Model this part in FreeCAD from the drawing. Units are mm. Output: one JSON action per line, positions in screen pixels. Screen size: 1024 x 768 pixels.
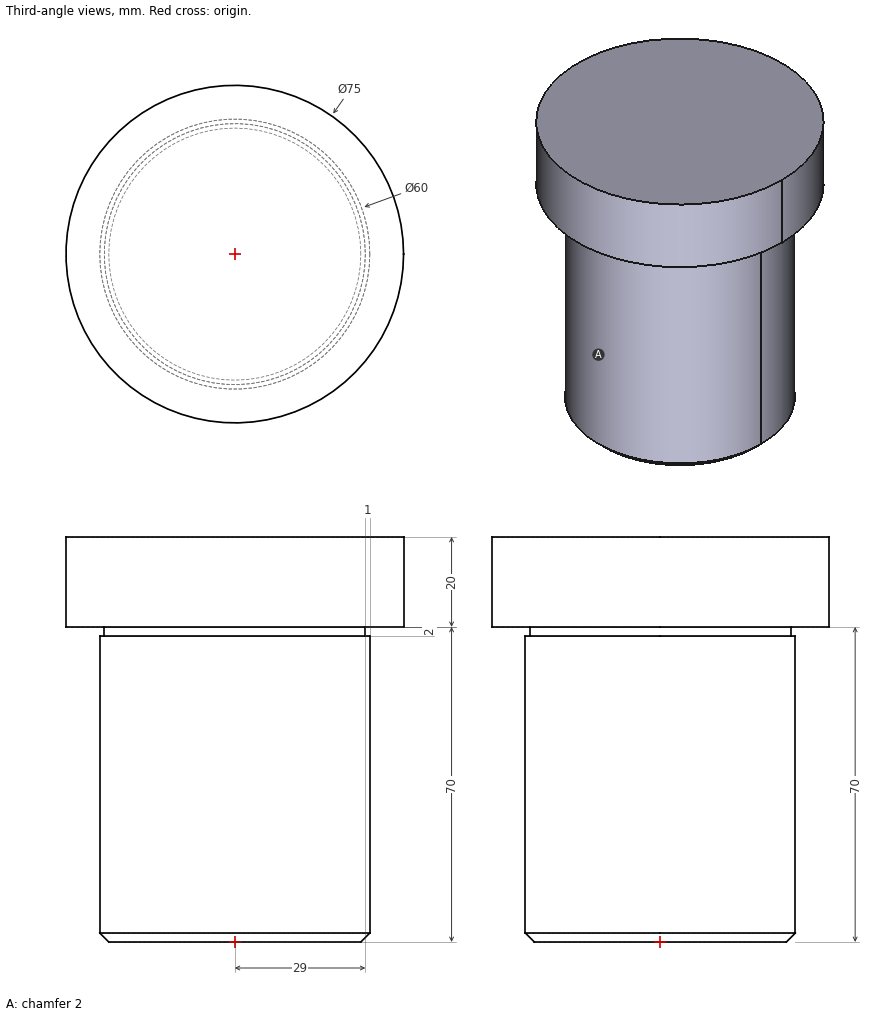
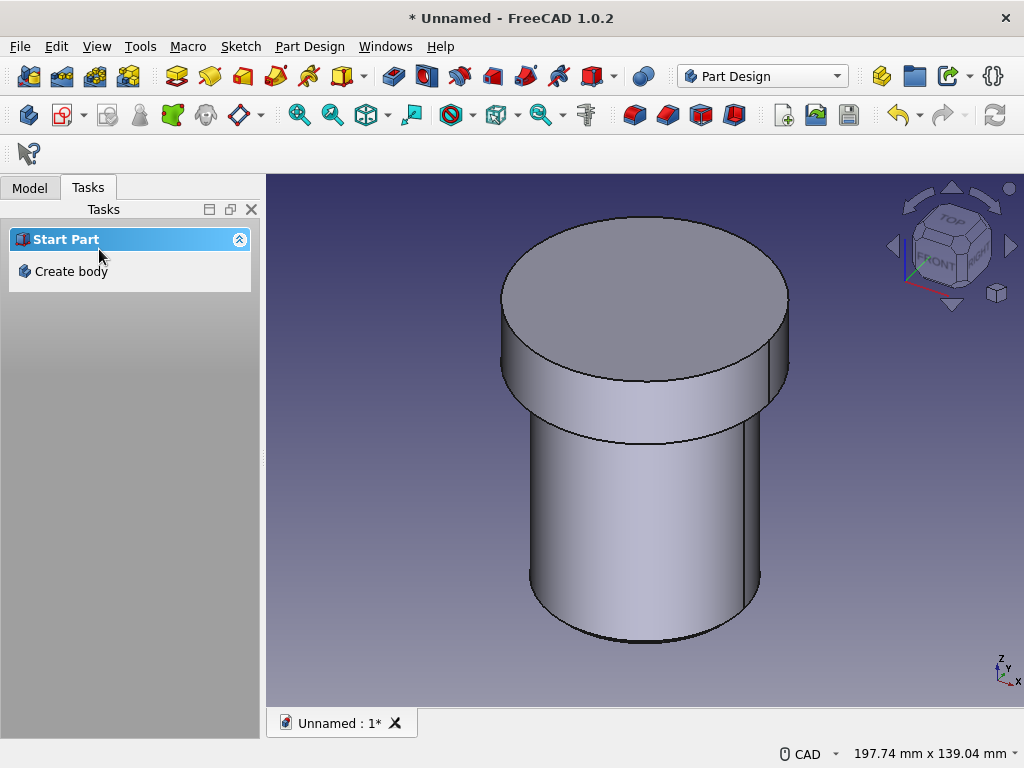
{"action": "left_click", "coordinate": [62, 116]}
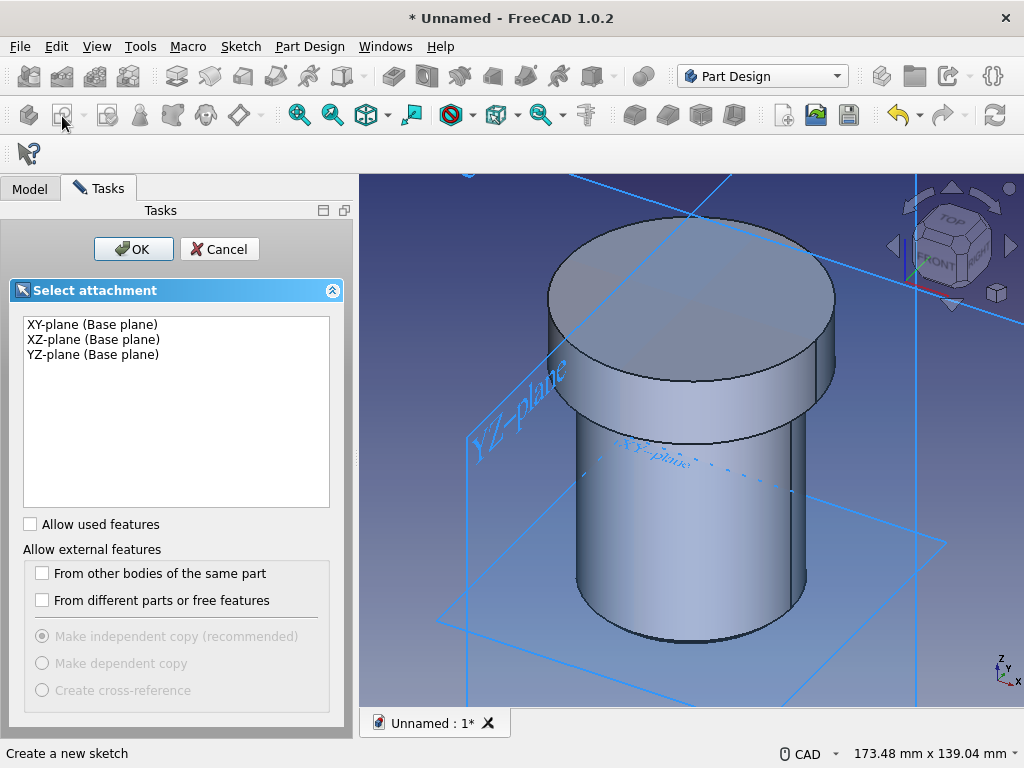
{"action": "left_click", "coordinate": [84, 340]}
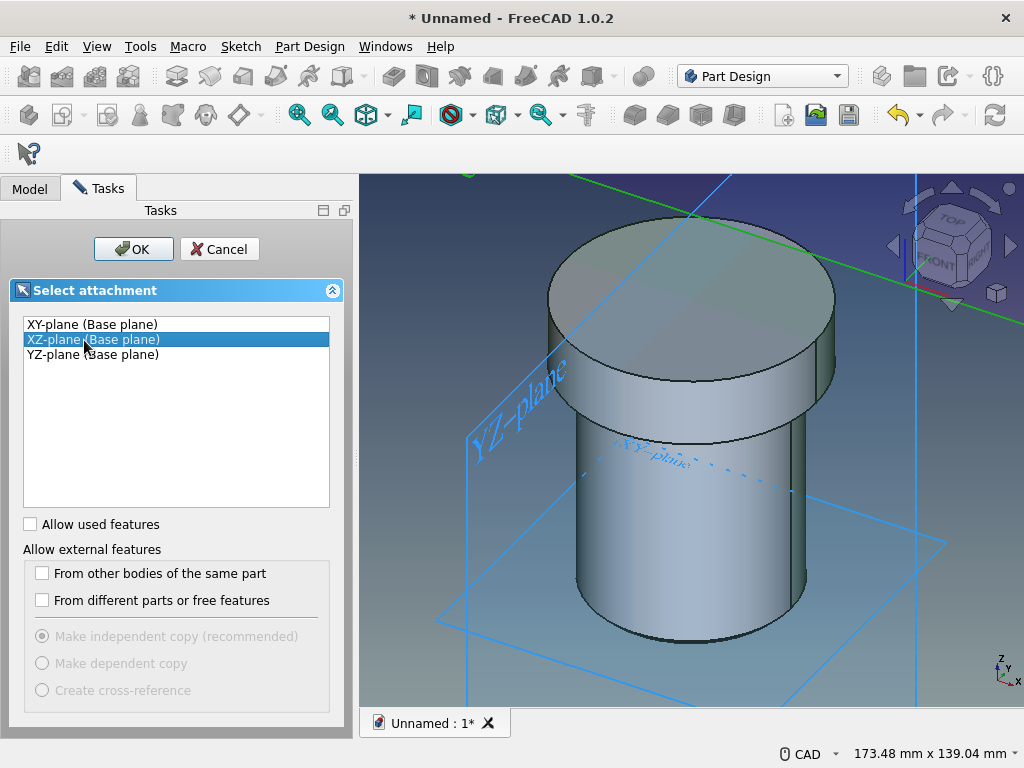
{"action": "left_click", "coordinate": [134, 249]}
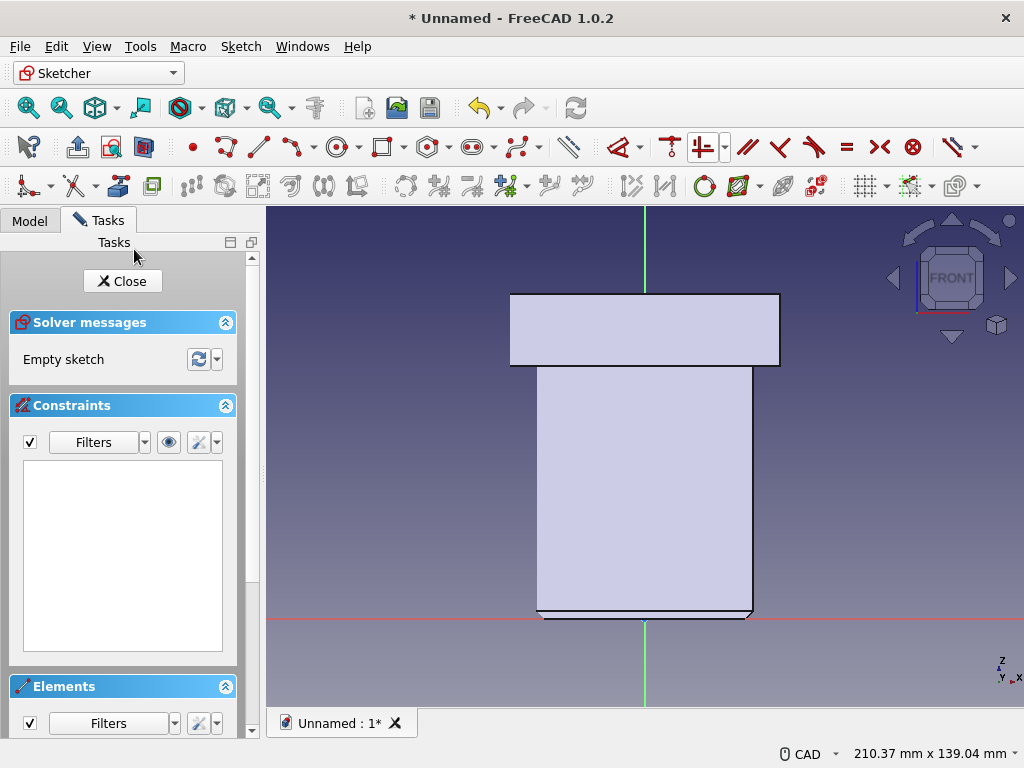
{"action": "left_click", "coordinate": [144, 148]}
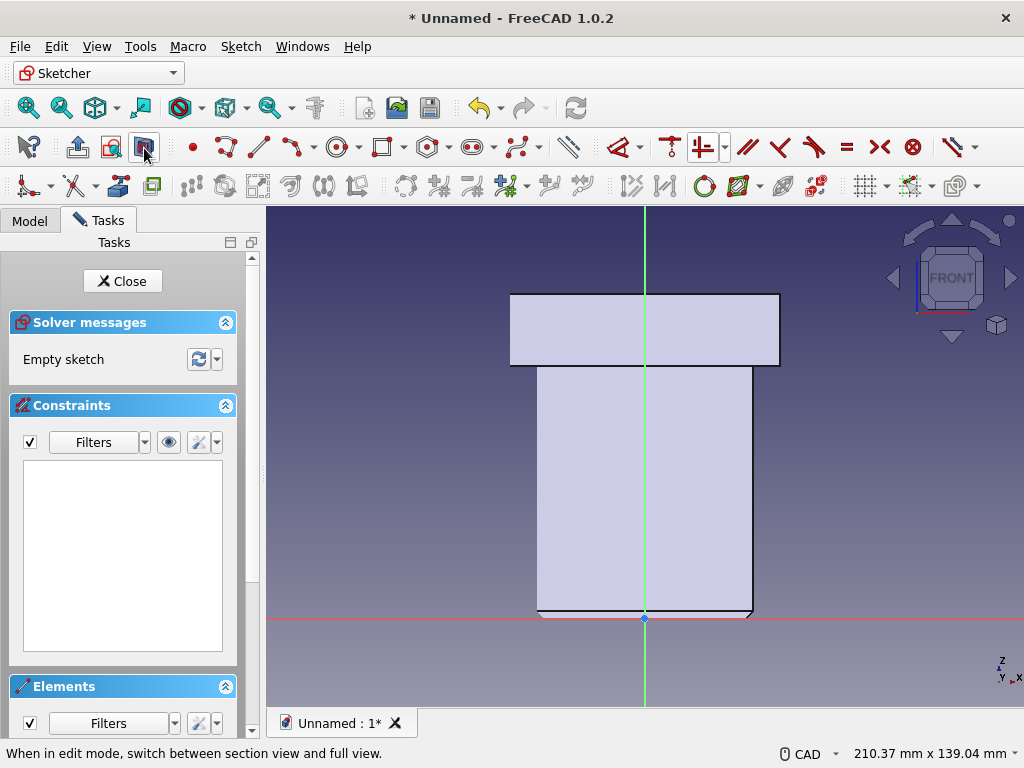
{"action": "scroll", "coordinate": [760, 365], "scroll_direction": "up", "scroll_amount": 15}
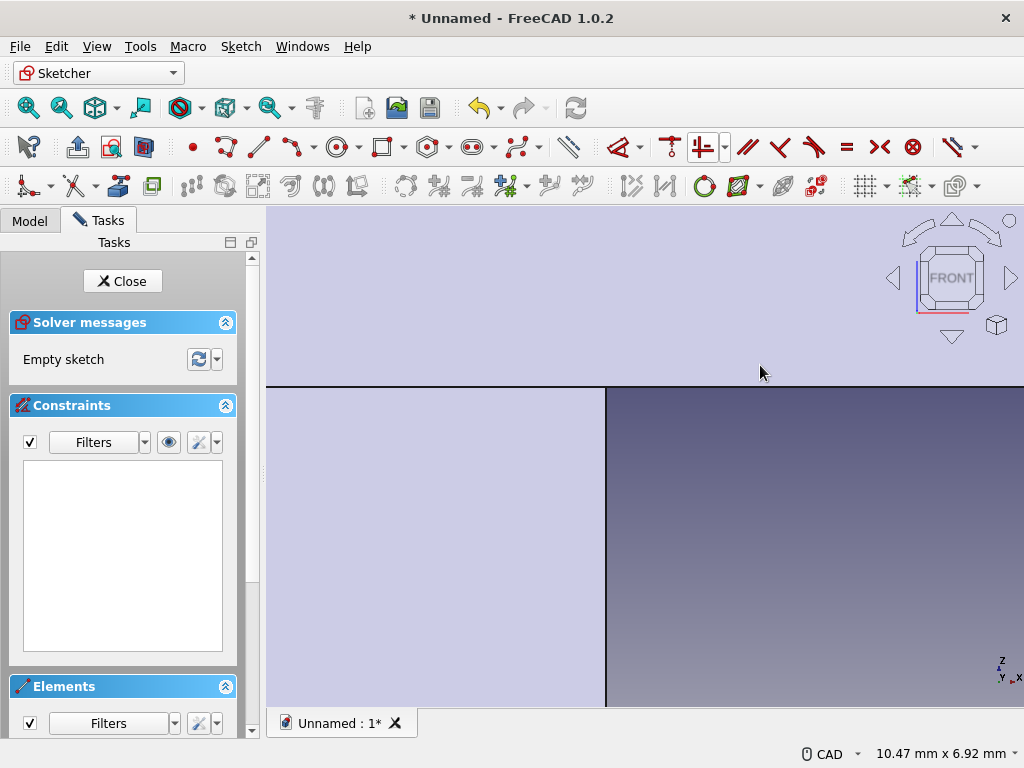
{"action": "scroll", "coordinate": [565, 463], "scroll_direction": "up", "scroll_amount": 4}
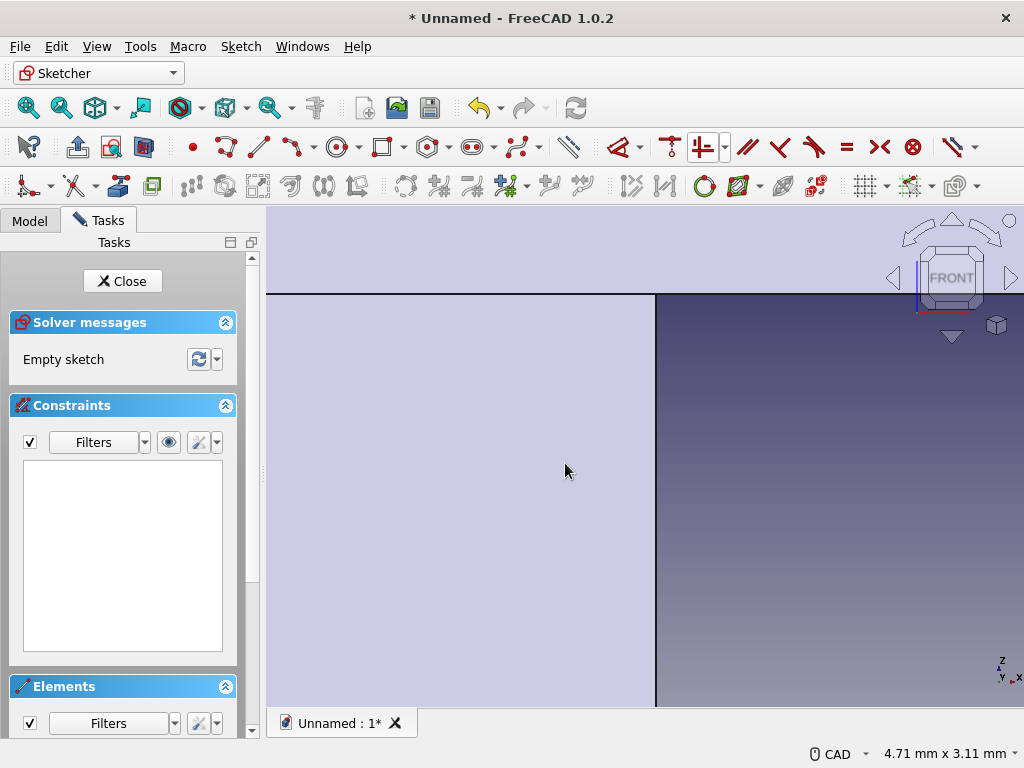
{"action": "key", "text": "g r"}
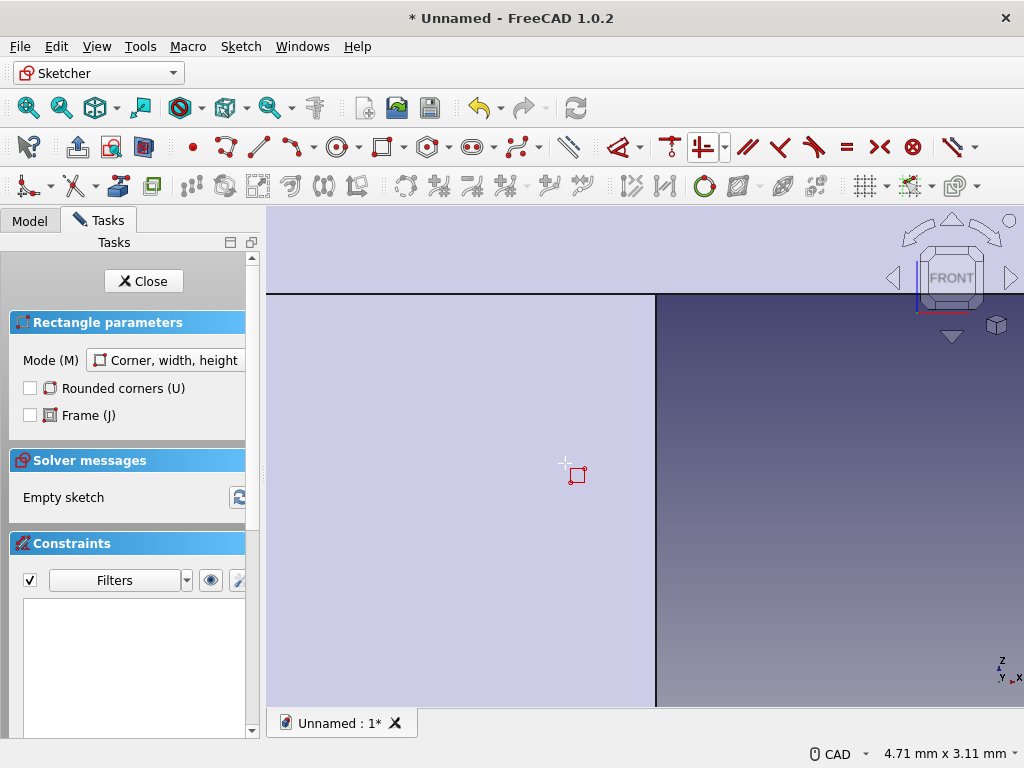
{"action": "left_click", "coordinate": [495, 294]}
{"action": "mouse_move", "coordinate": [656, 616]}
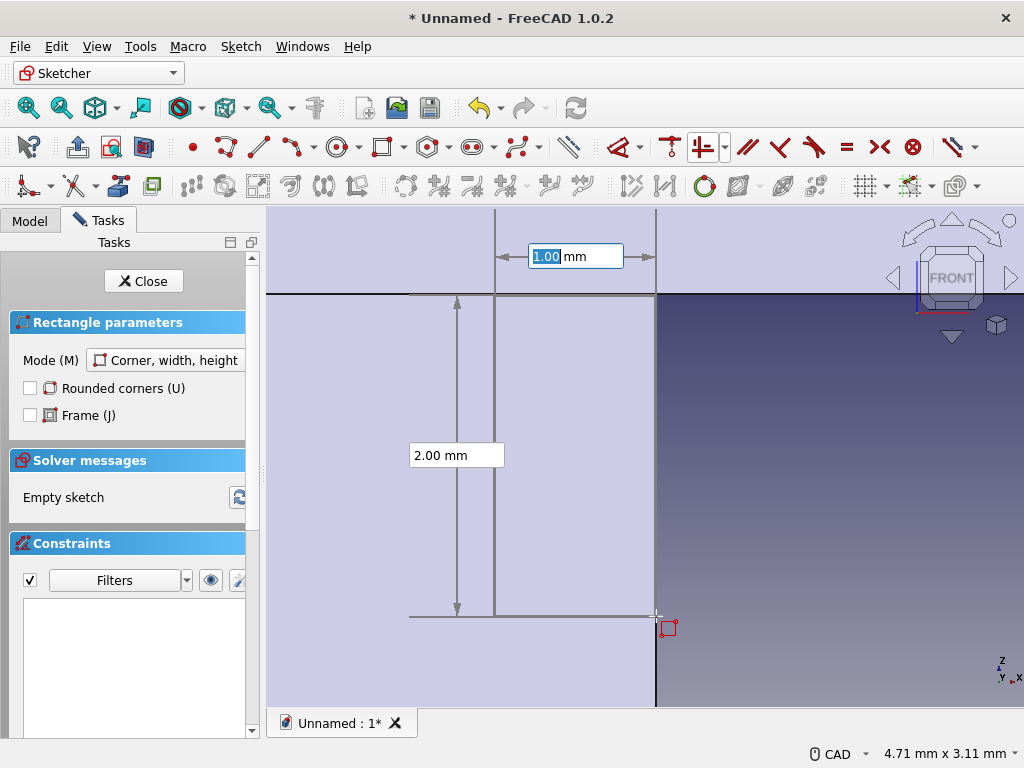
{"action": "type", "text": "1"}
{"action": "key", "text": "Tab"}
{"action": "type", "text": "2"}
{"action": "key", "text": "Return"}
{"action": "key", "text": "Escape"}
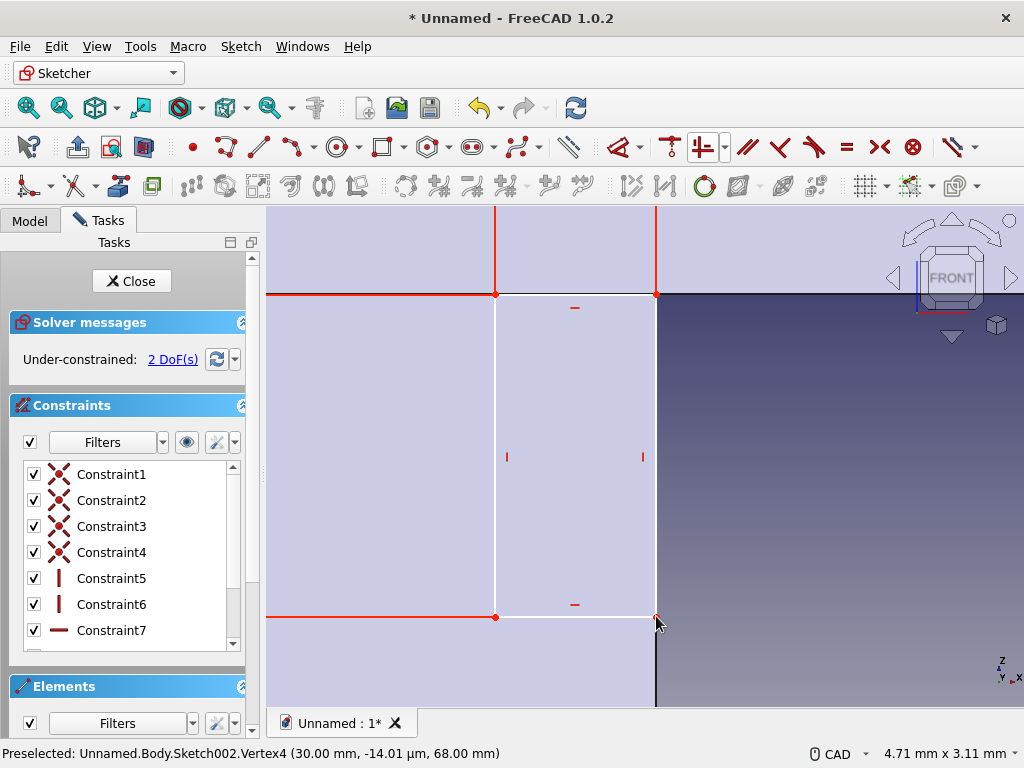
{"action": "left_click", "coordinate": [495, 295]}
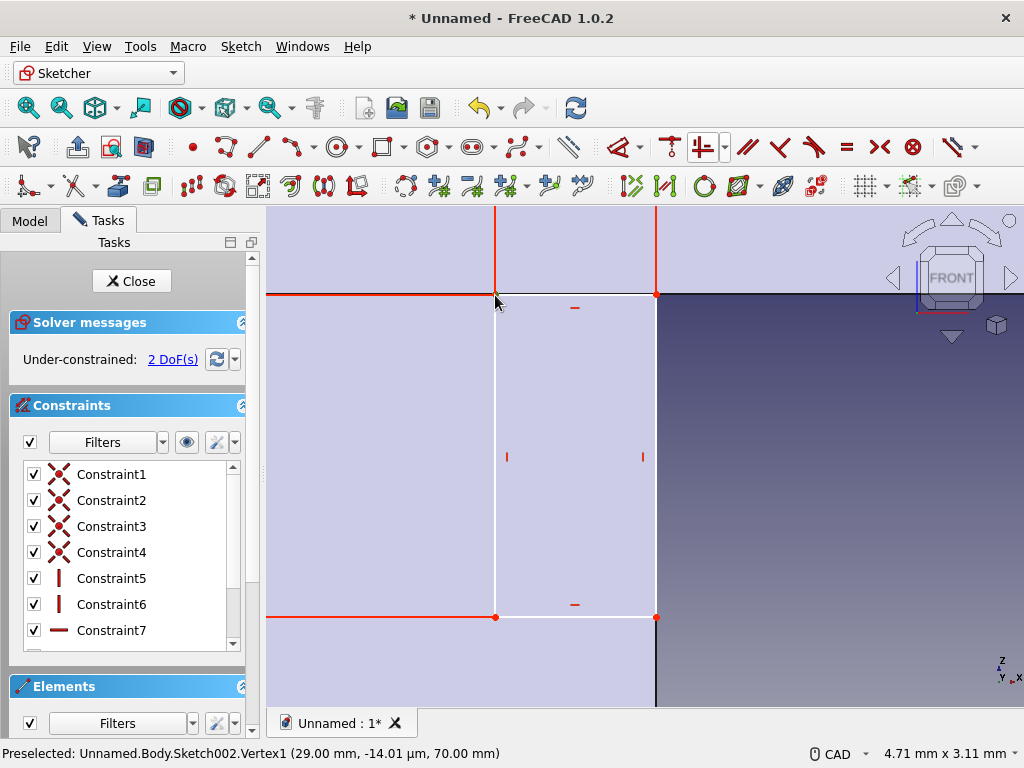
{"action": "key", "text": "l"}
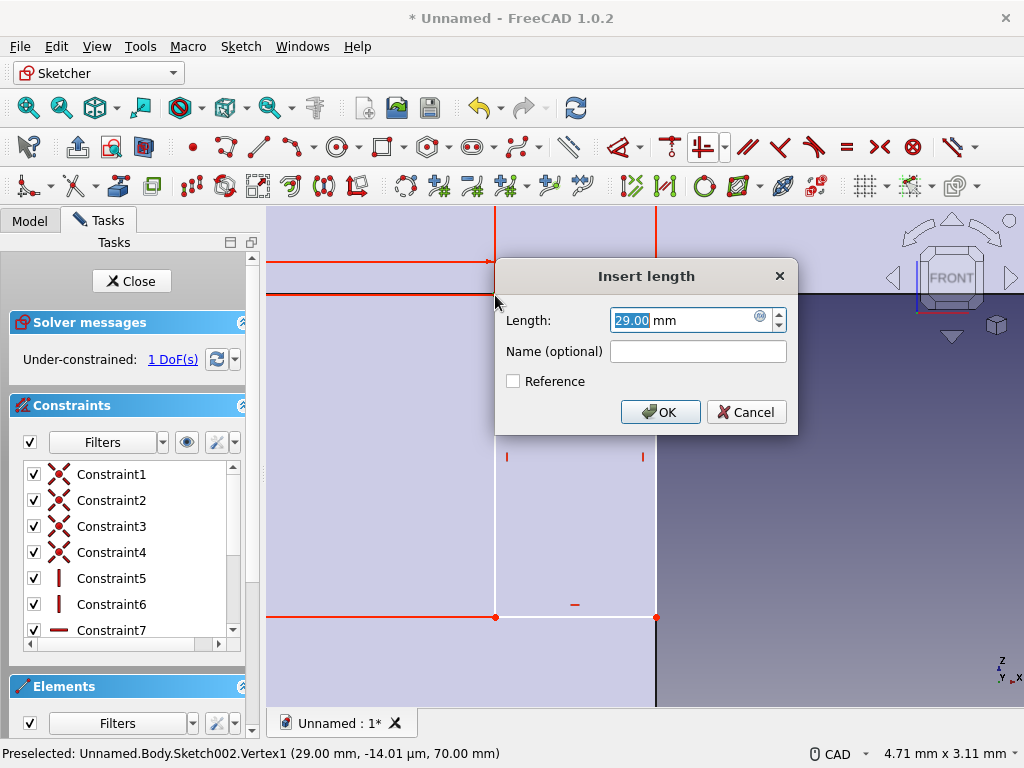
{"action": "type", "text": "29"}
{"action": "key", "text": "Return"}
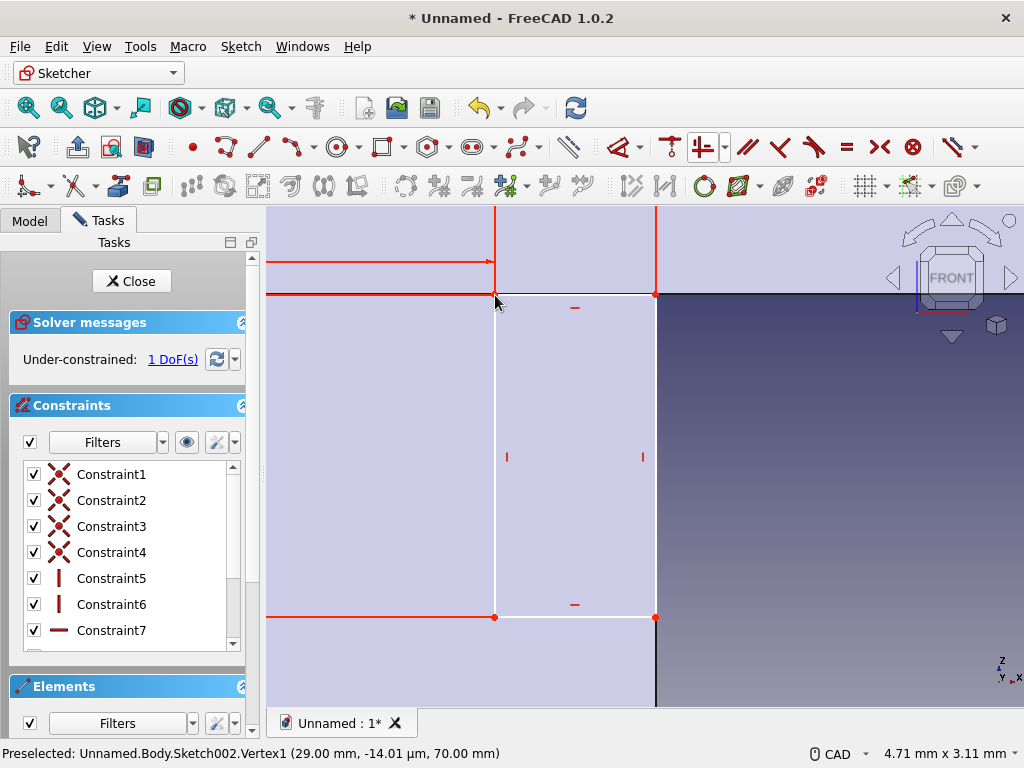
{"action": "left_click", "coordinate": [495, 295]}